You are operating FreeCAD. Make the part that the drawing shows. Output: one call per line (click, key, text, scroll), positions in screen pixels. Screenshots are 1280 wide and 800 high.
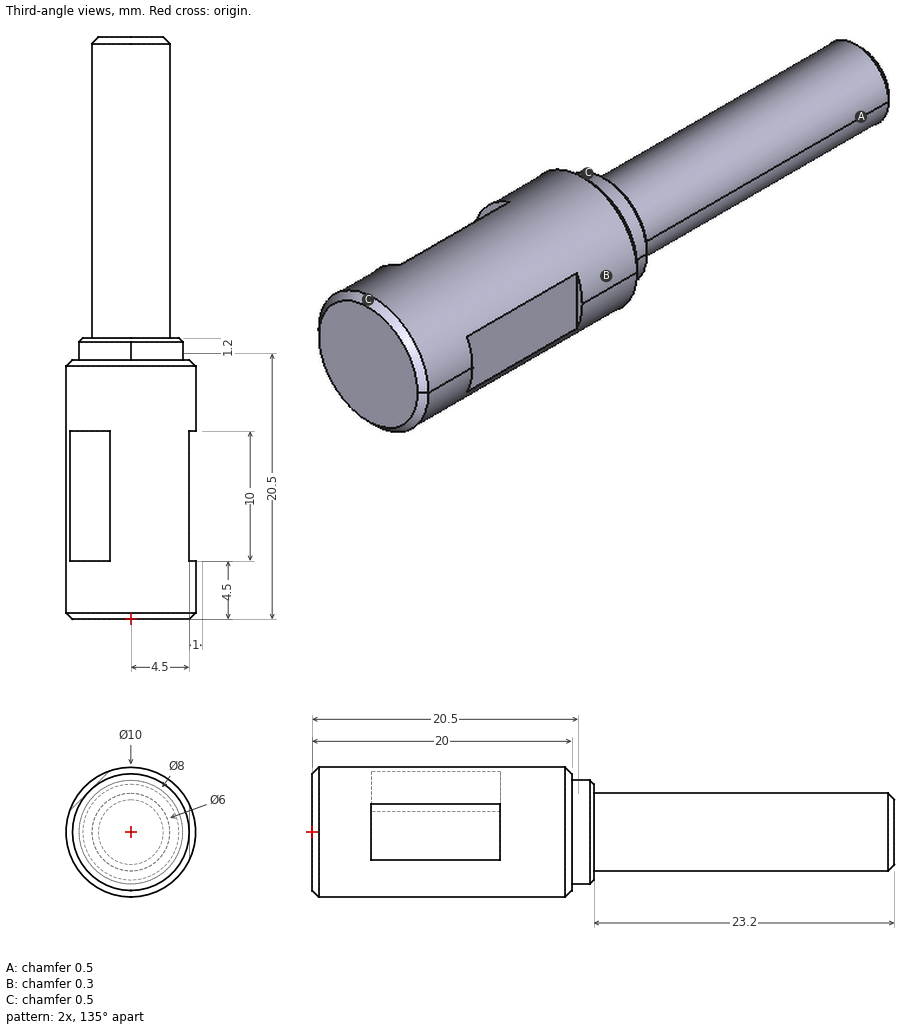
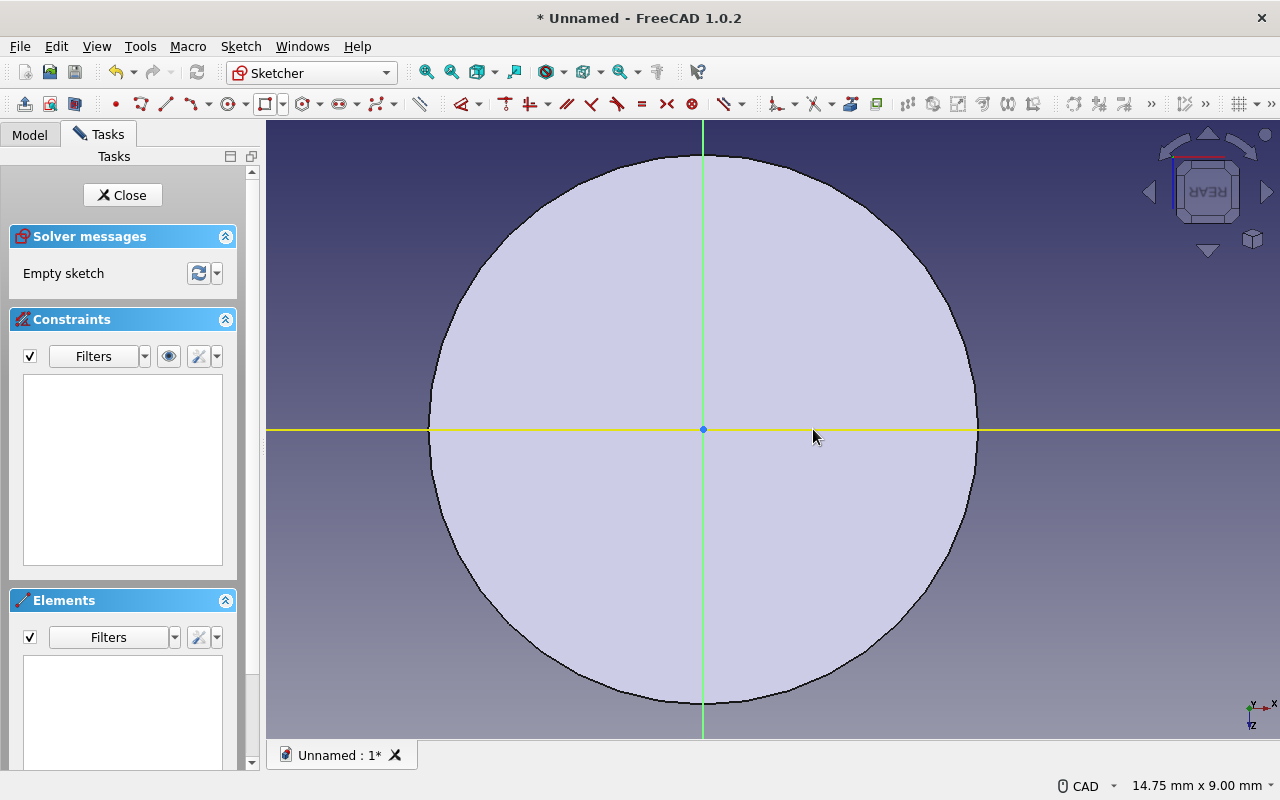
click(228, 104)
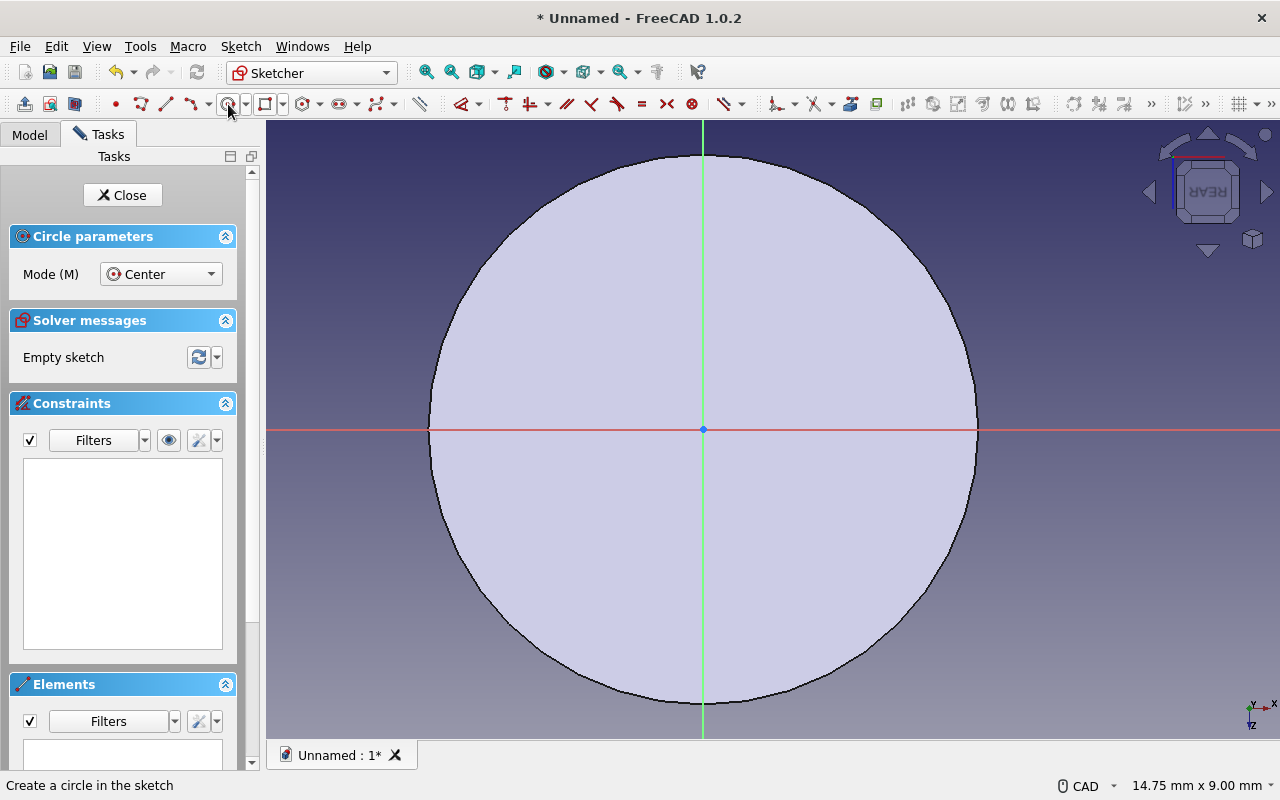
click(703, 429)
move(849, 284)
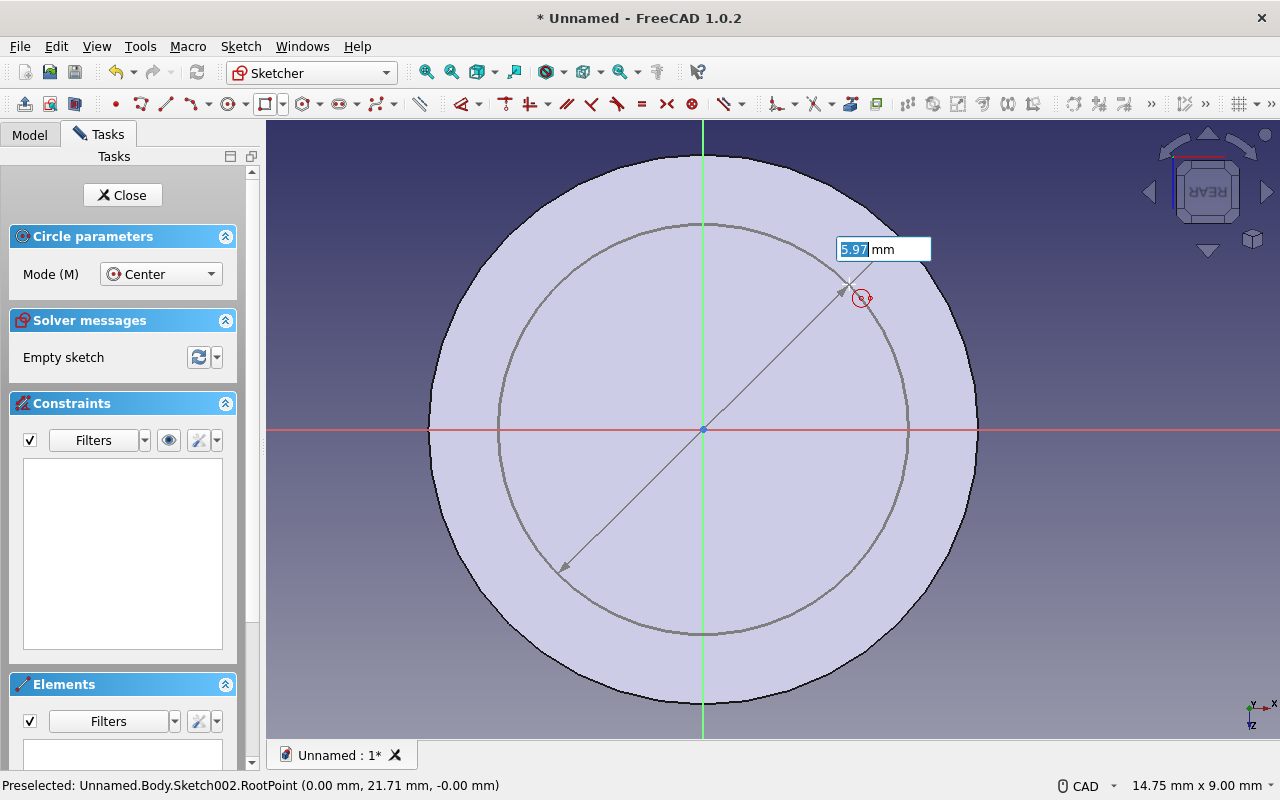
text(6)
key(Return)
key(Escape)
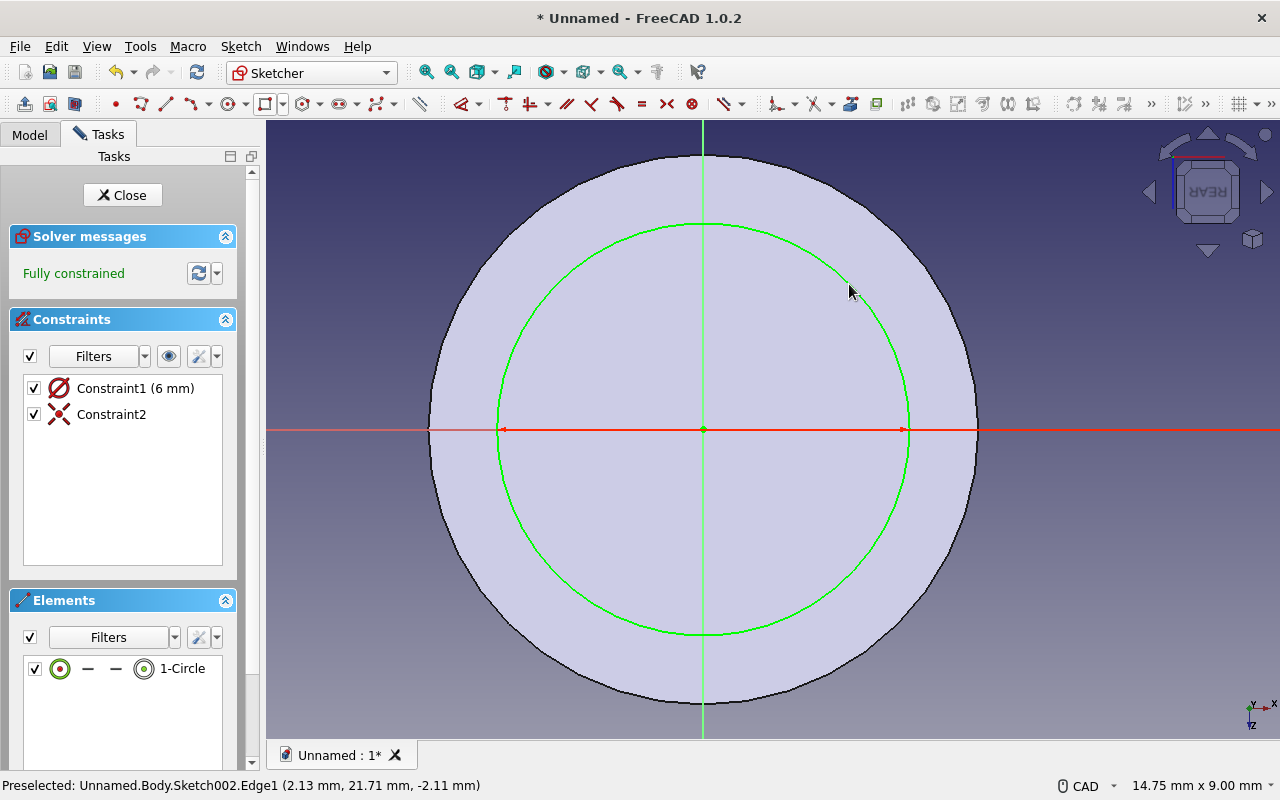
click(123, 195)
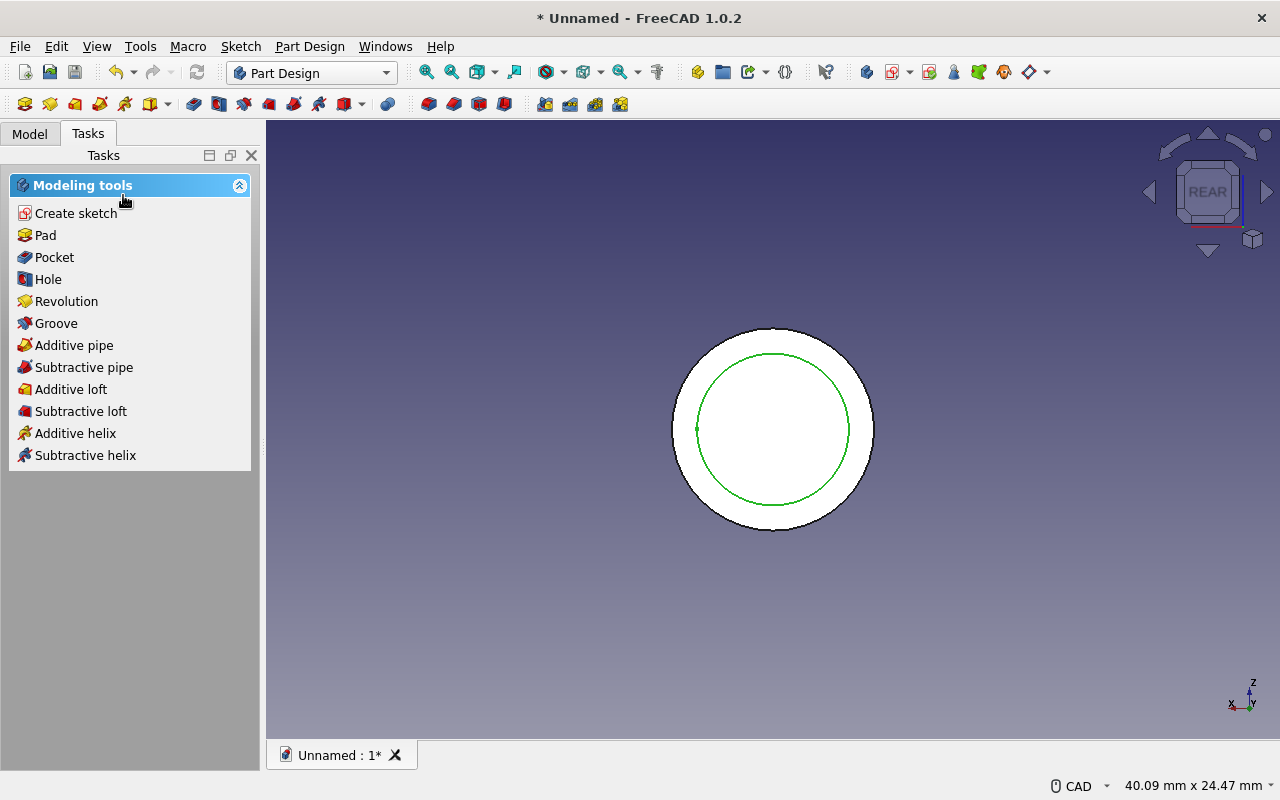
click(25, 104)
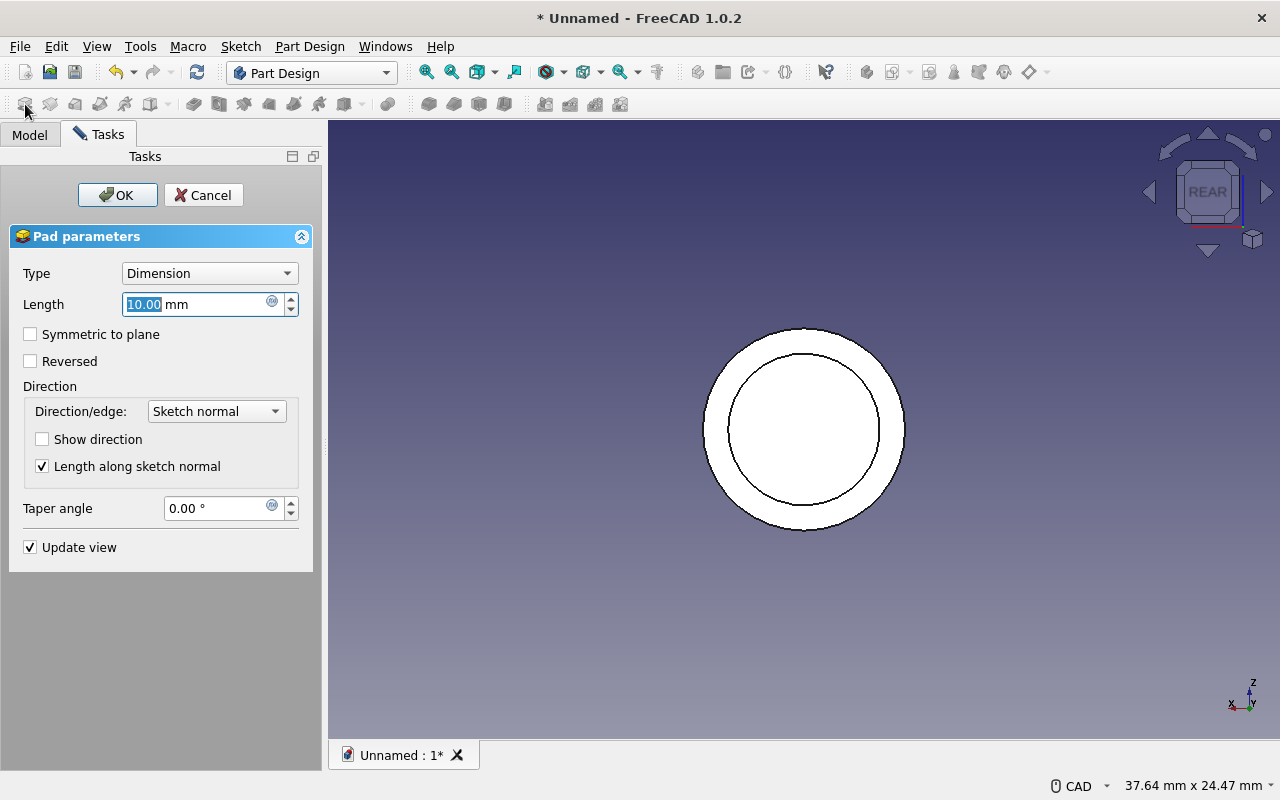
text(23.2)
key(Tab)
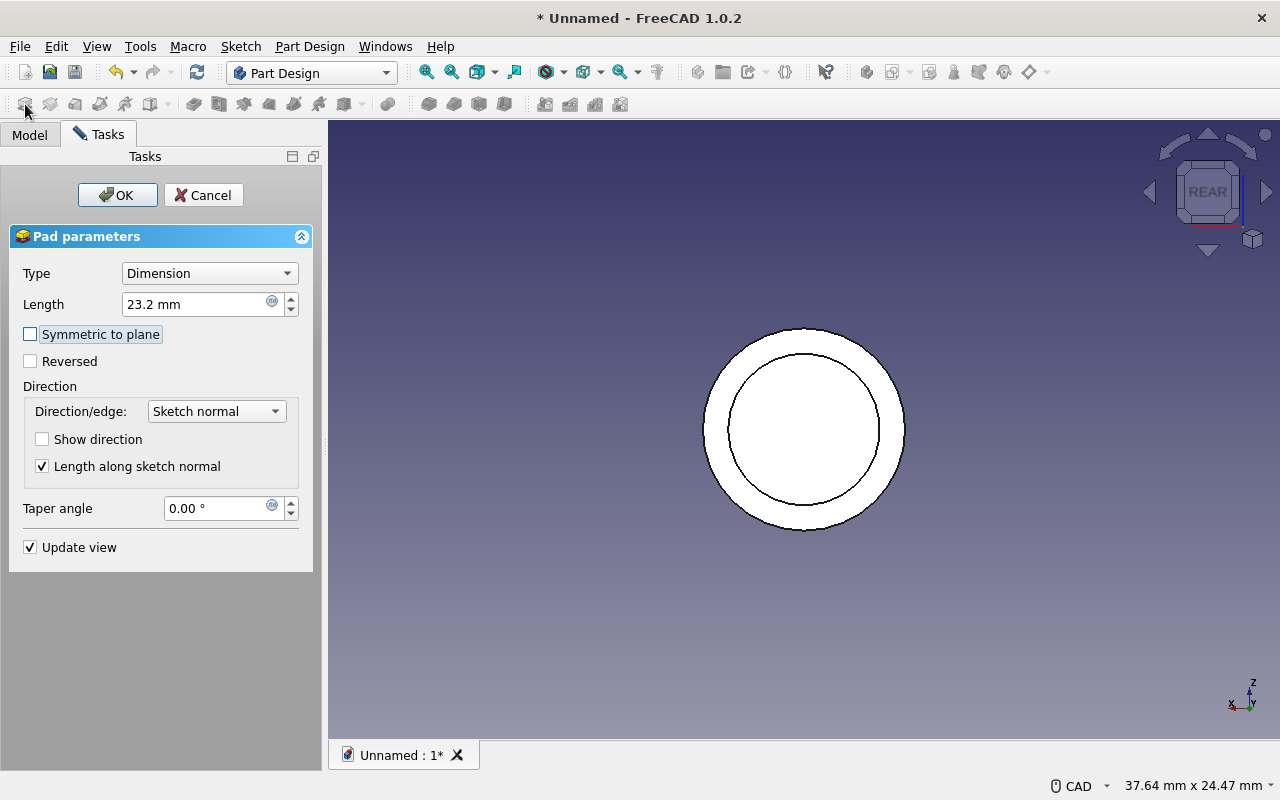
click(118, 195)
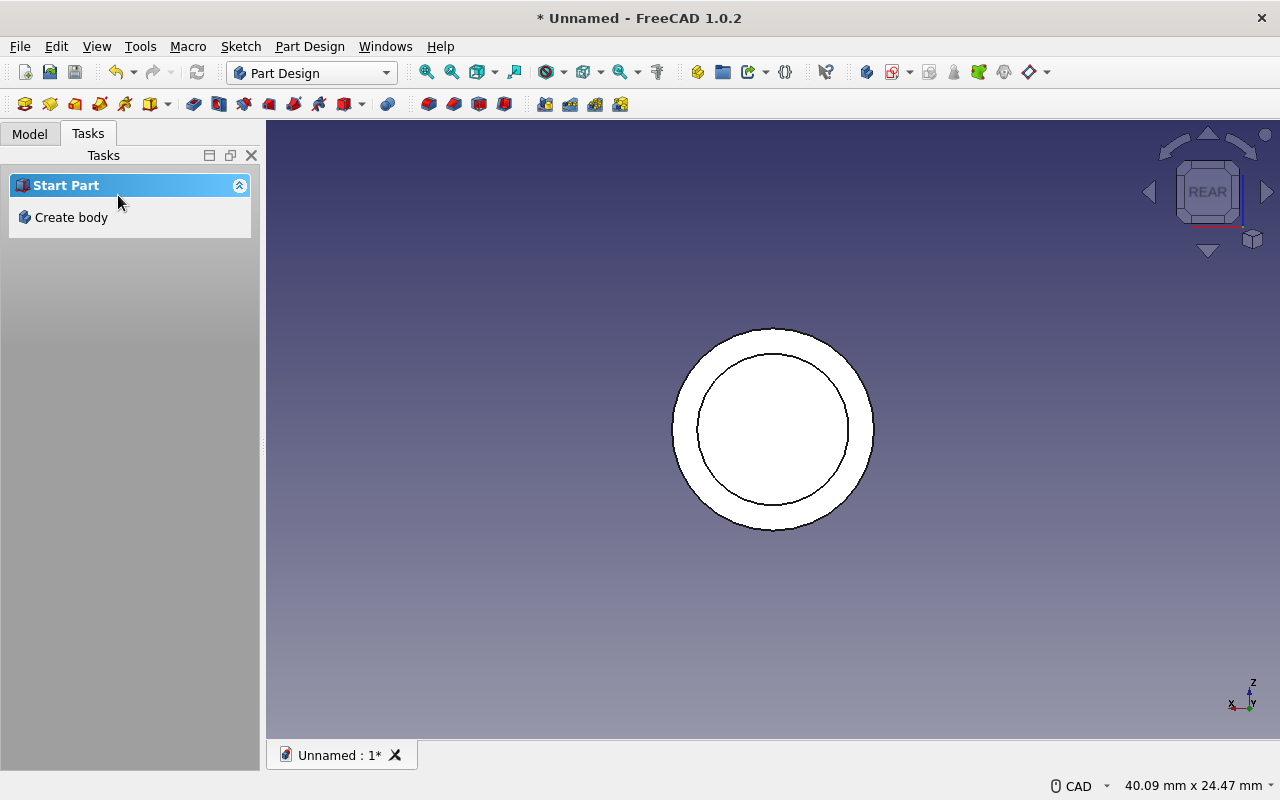
click(427, 72)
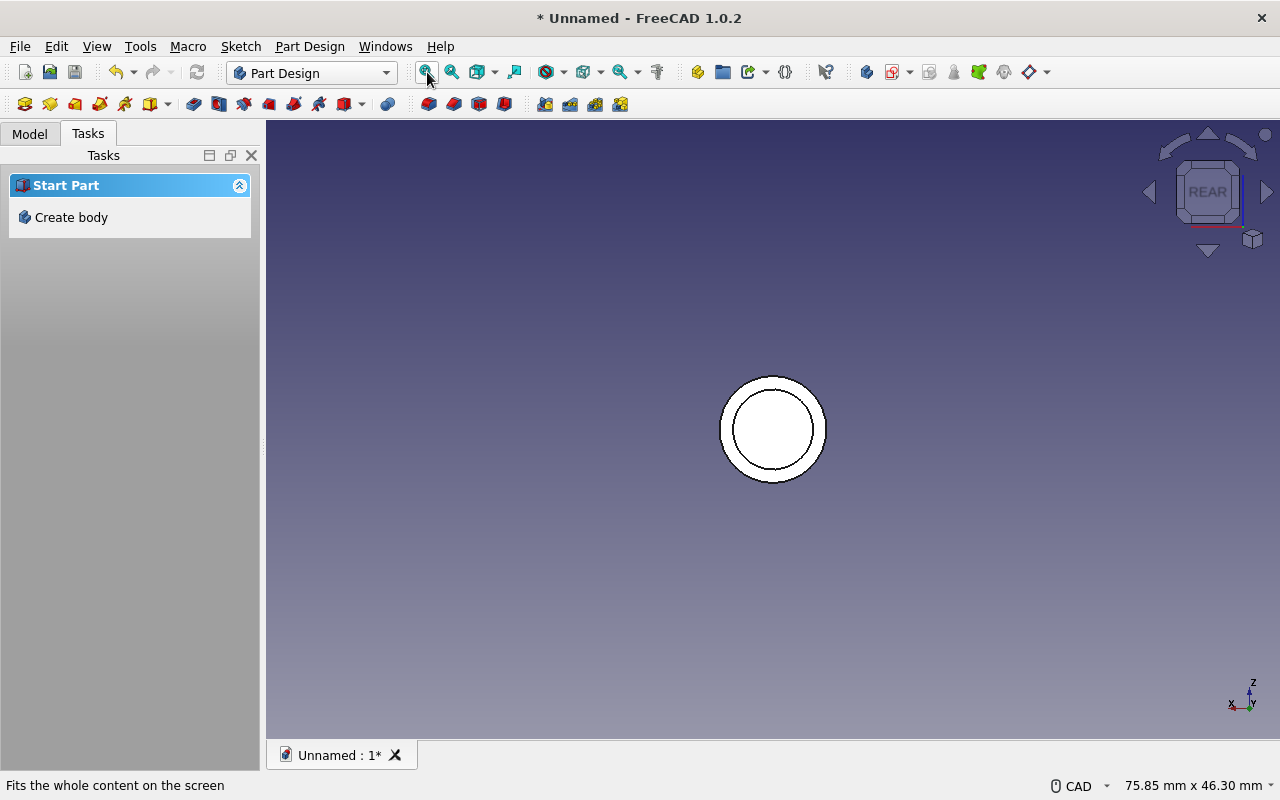
click(813, 428)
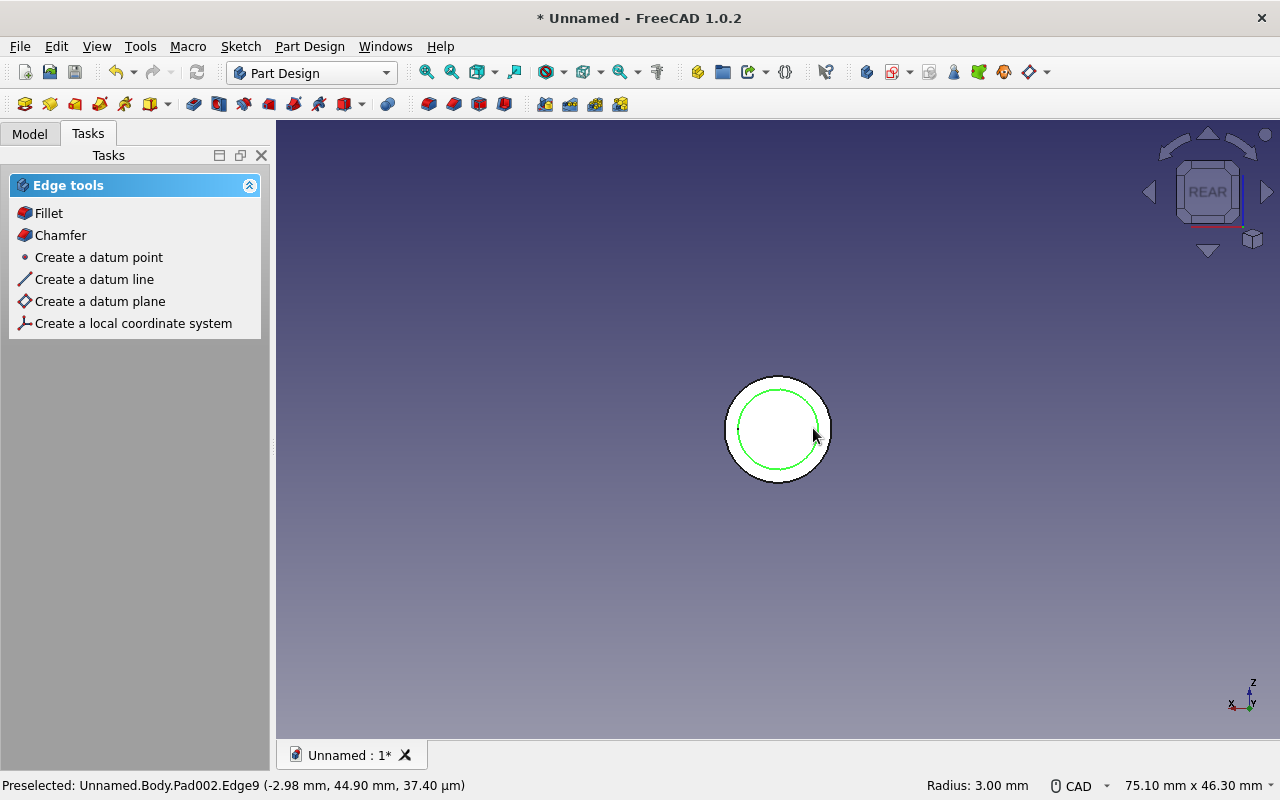
click(454, 104)